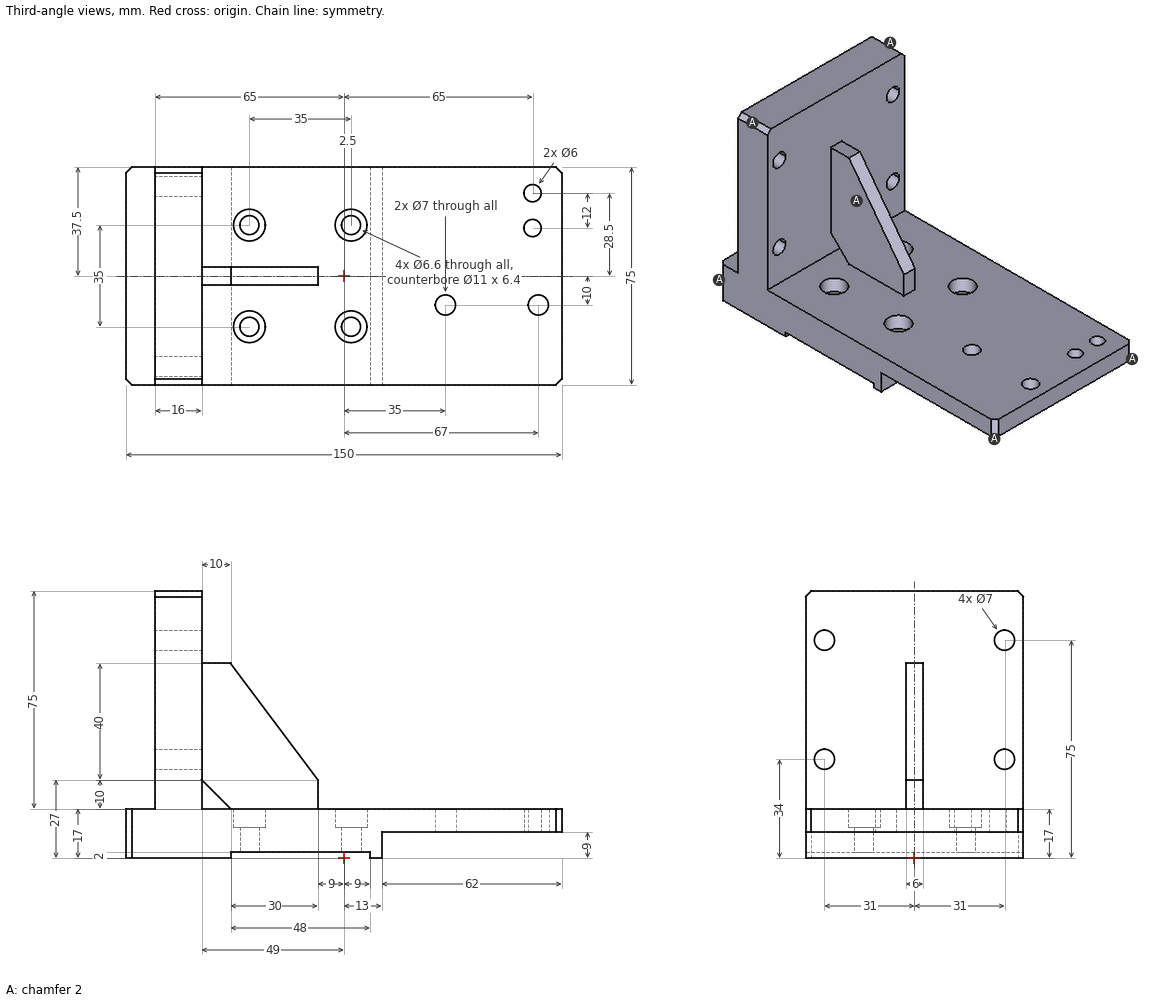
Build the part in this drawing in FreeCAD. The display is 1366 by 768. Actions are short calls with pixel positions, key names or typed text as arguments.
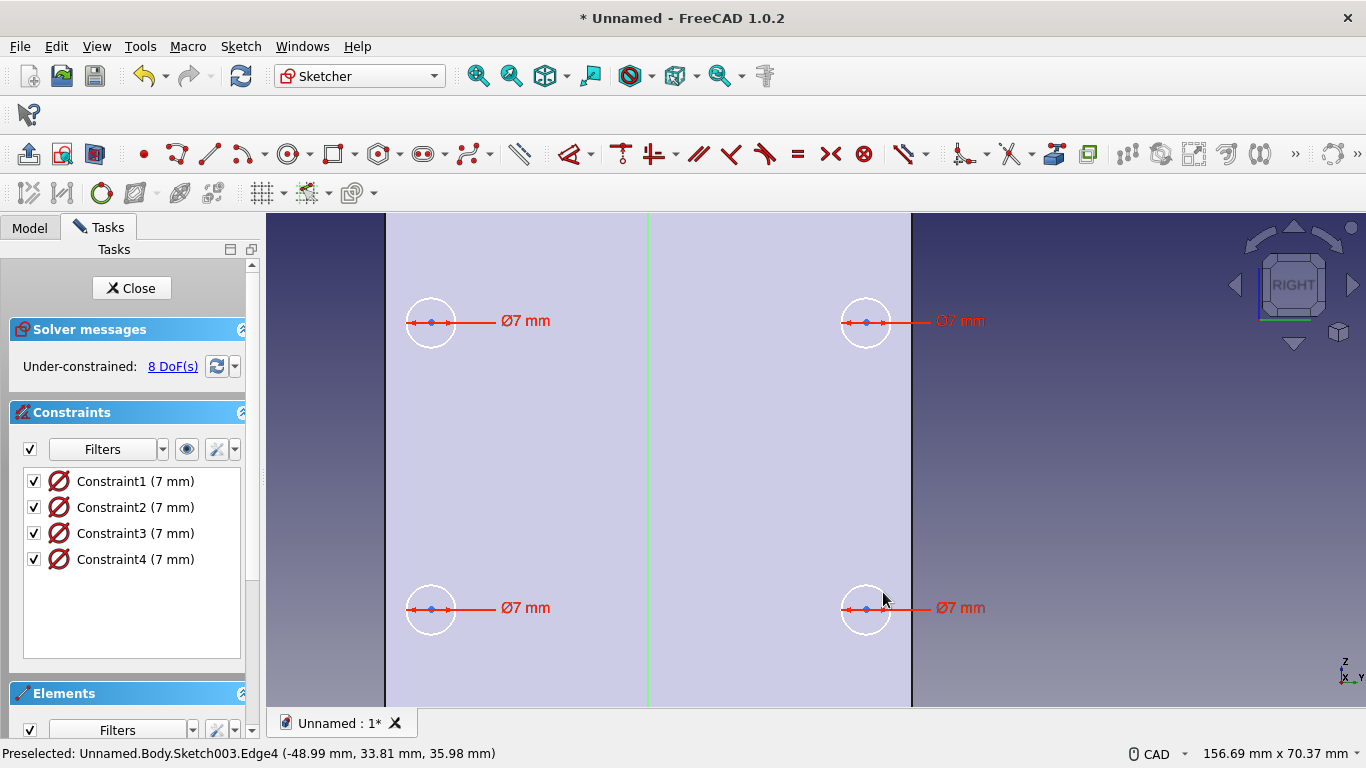
click(866, 323)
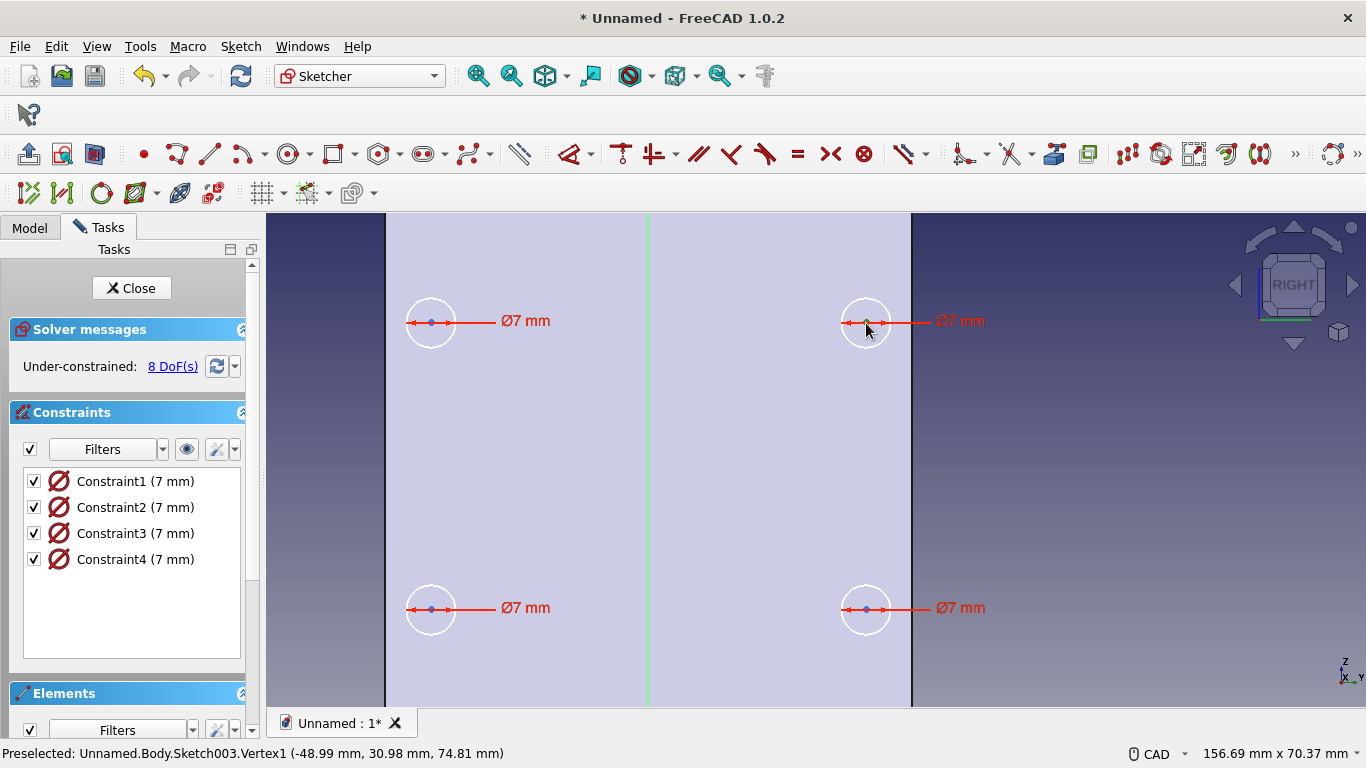
click(431, 323)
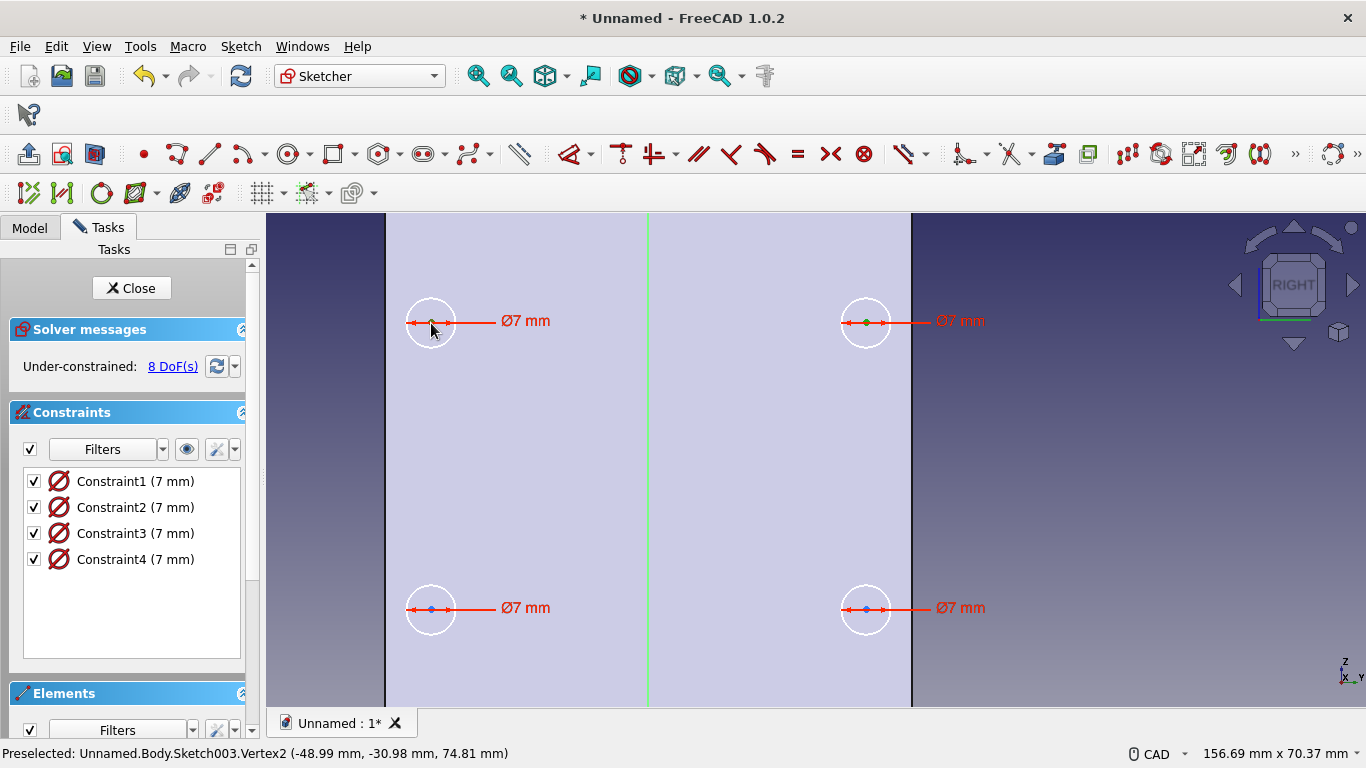
click(648, 648)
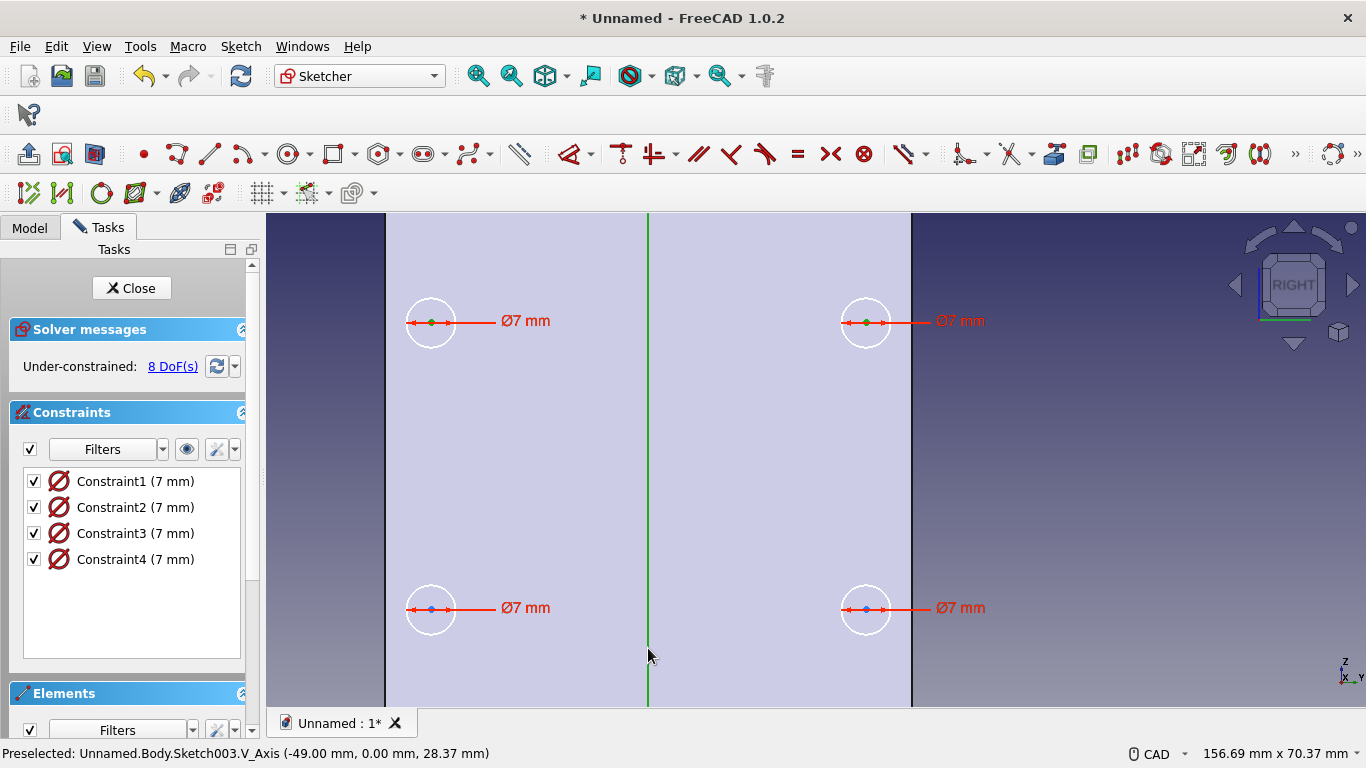
click(831, 154)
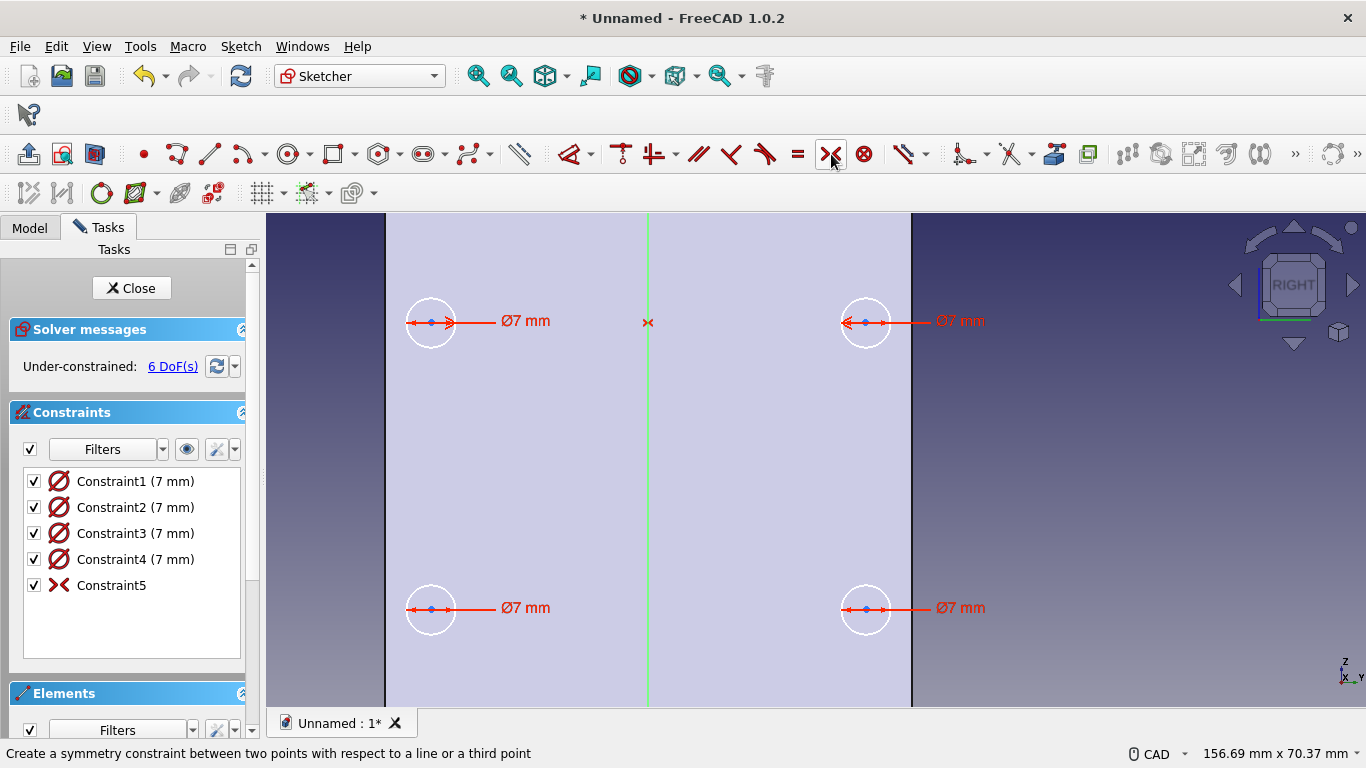
click(431, 610)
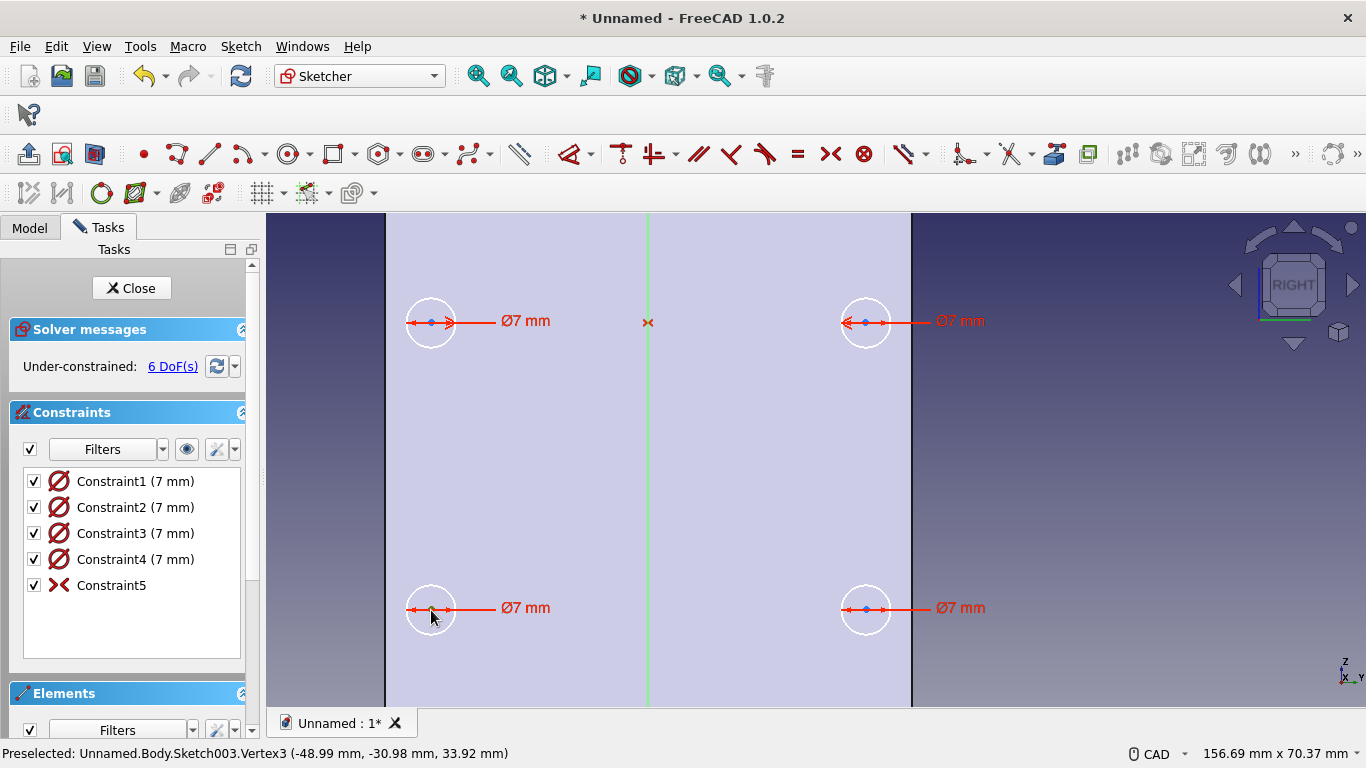
click(866, 610)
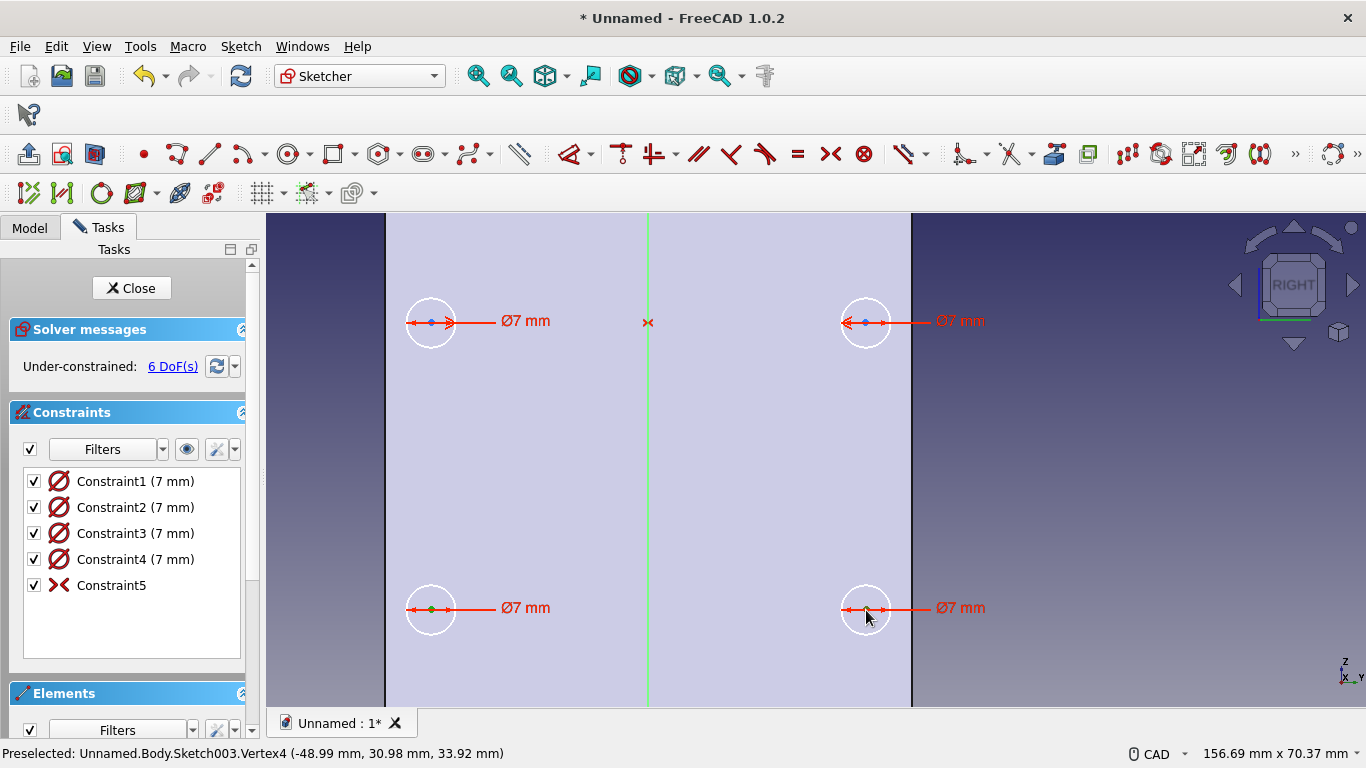
click(648, 648)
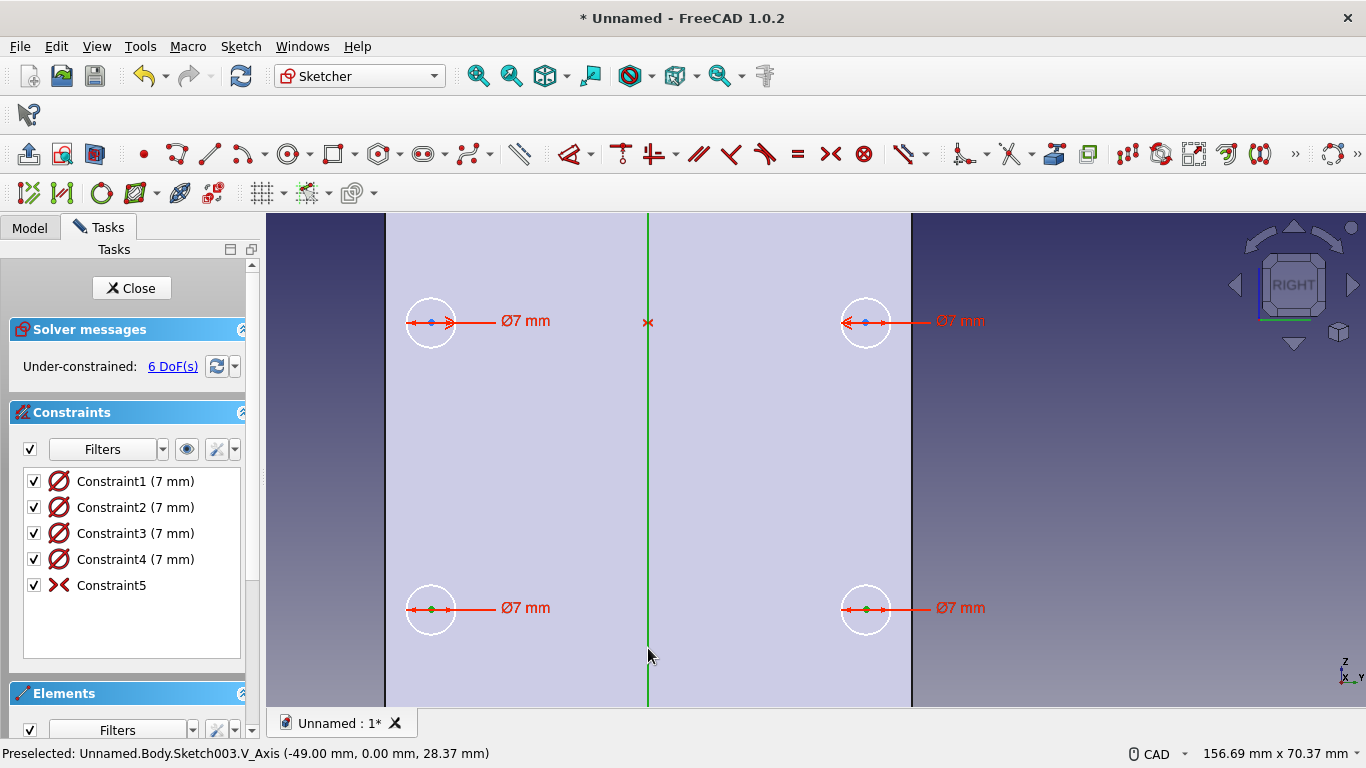
click(831, 154)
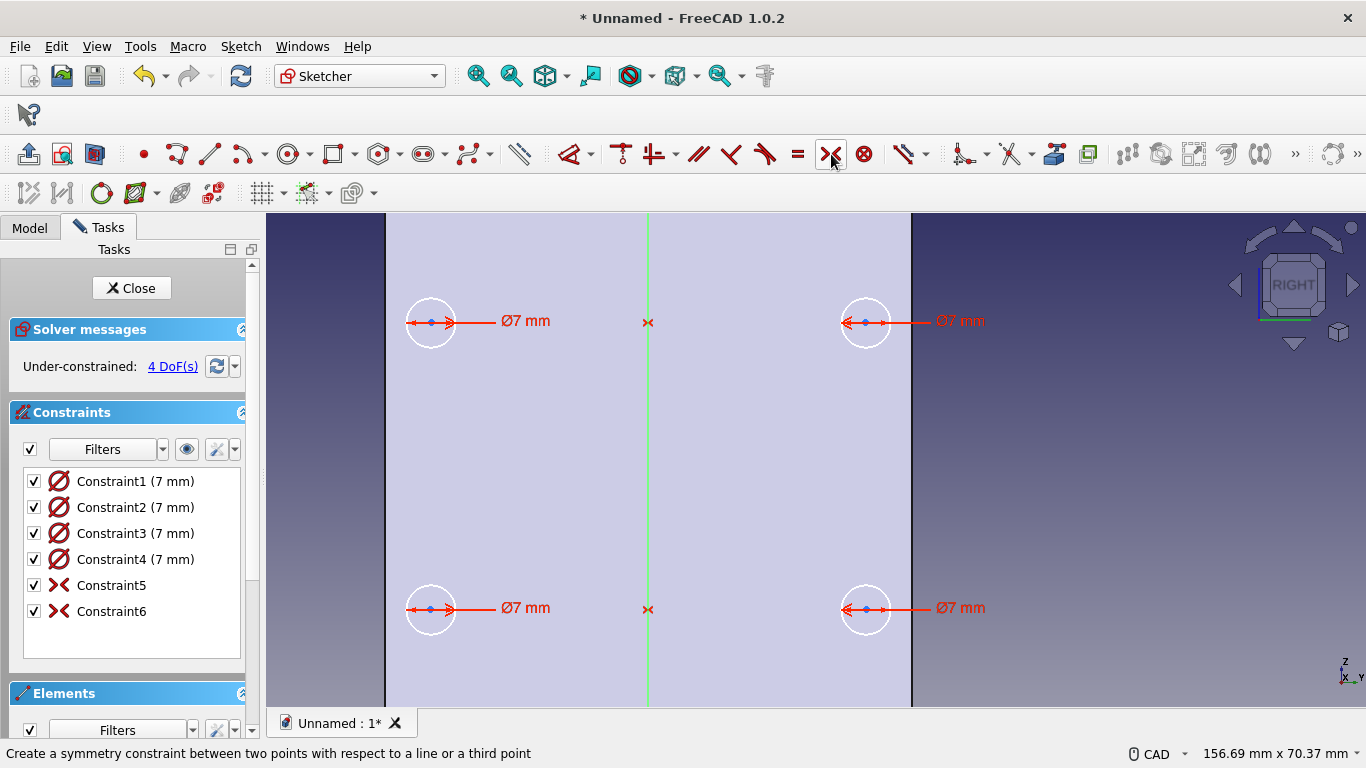
click(568, 154)